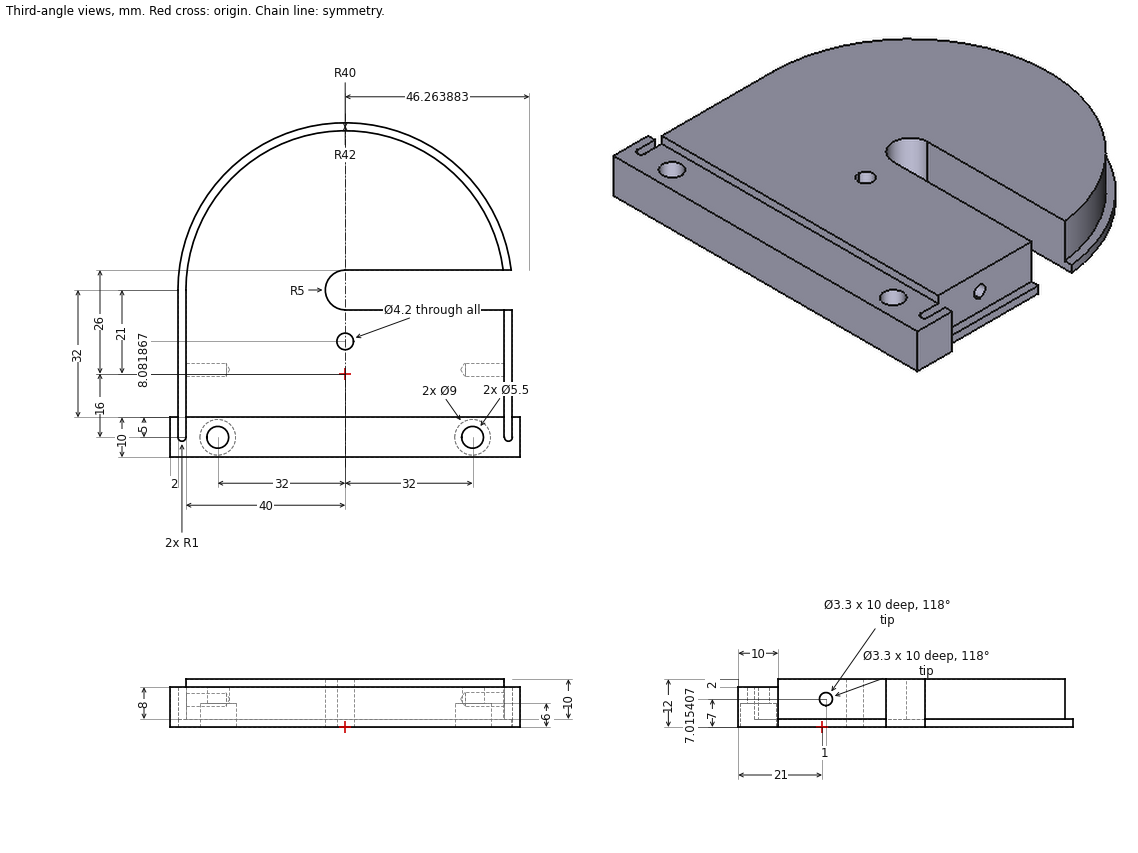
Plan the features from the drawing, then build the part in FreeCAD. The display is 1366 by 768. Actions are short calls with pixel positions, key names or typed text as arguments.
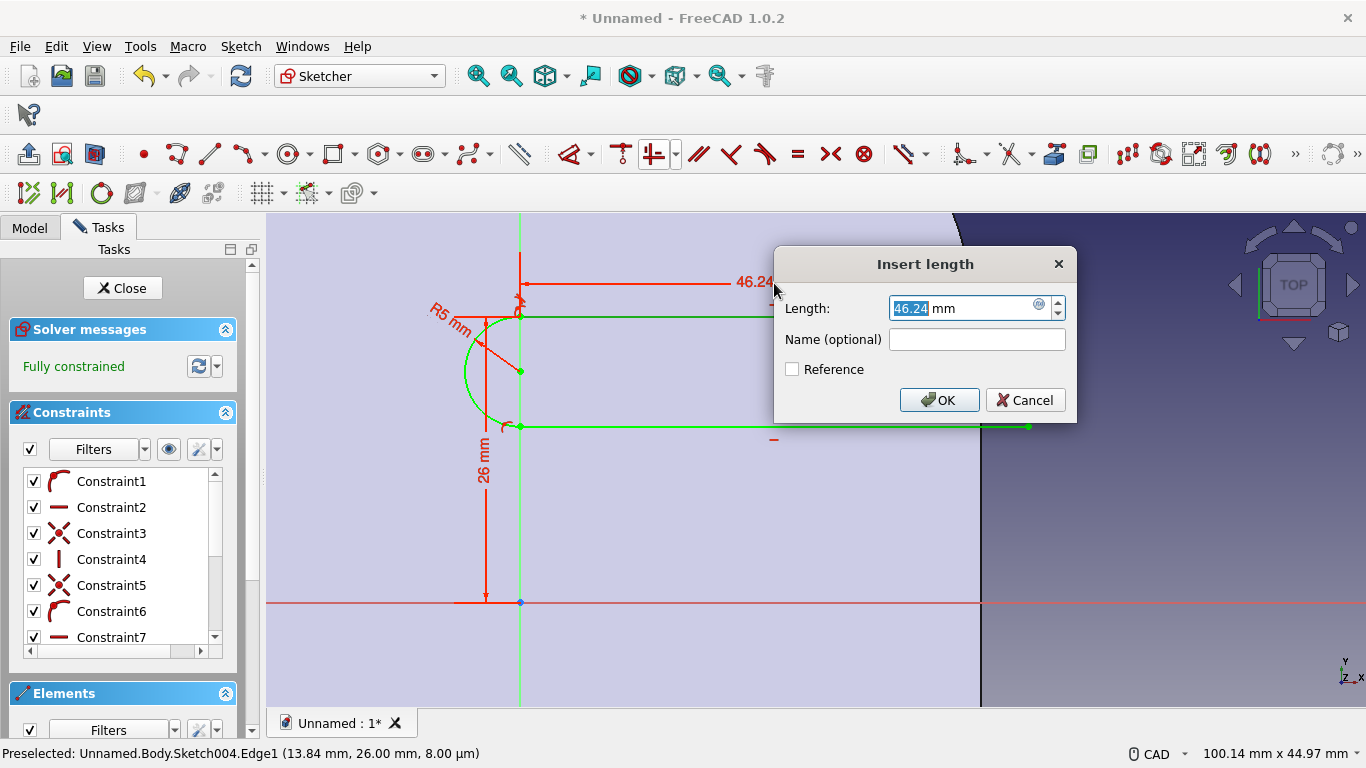
text(46.263883)
key(Return)
key(Escape)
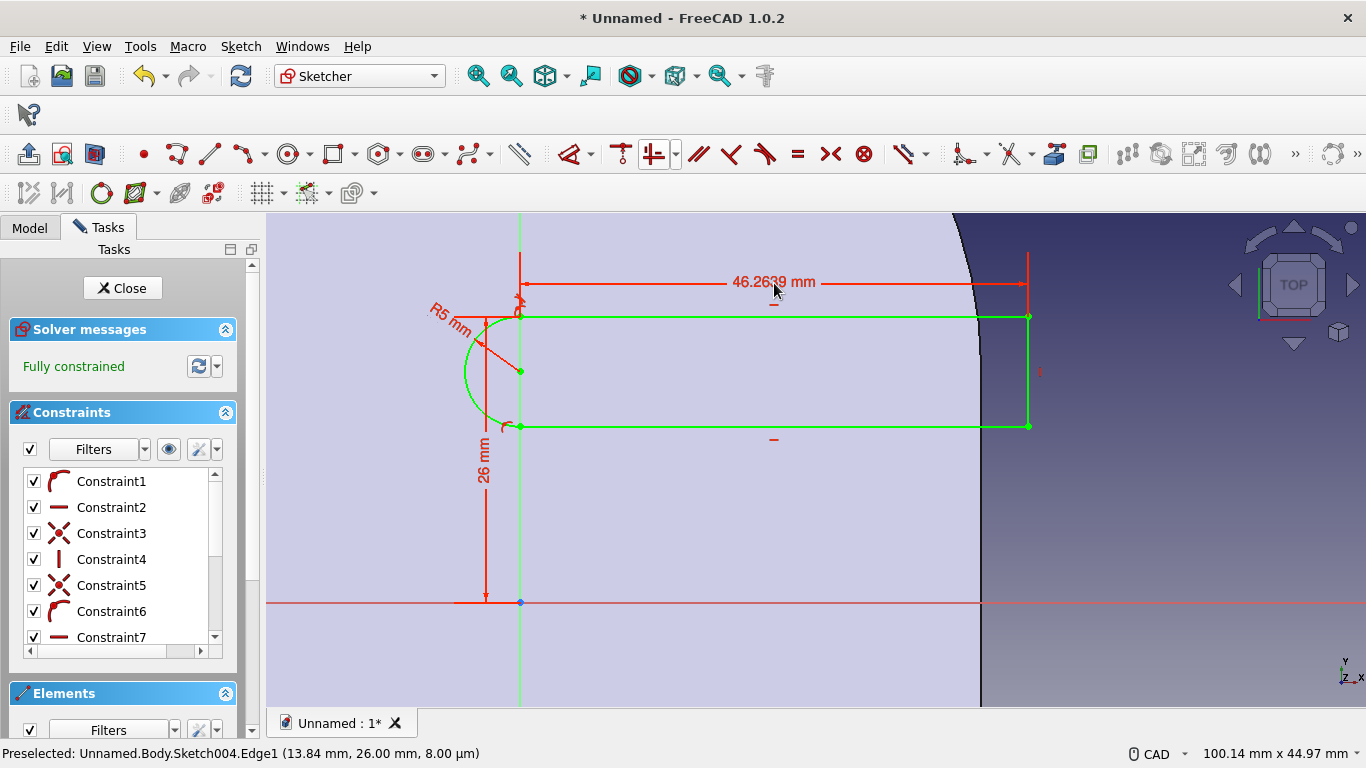
click(123, 288)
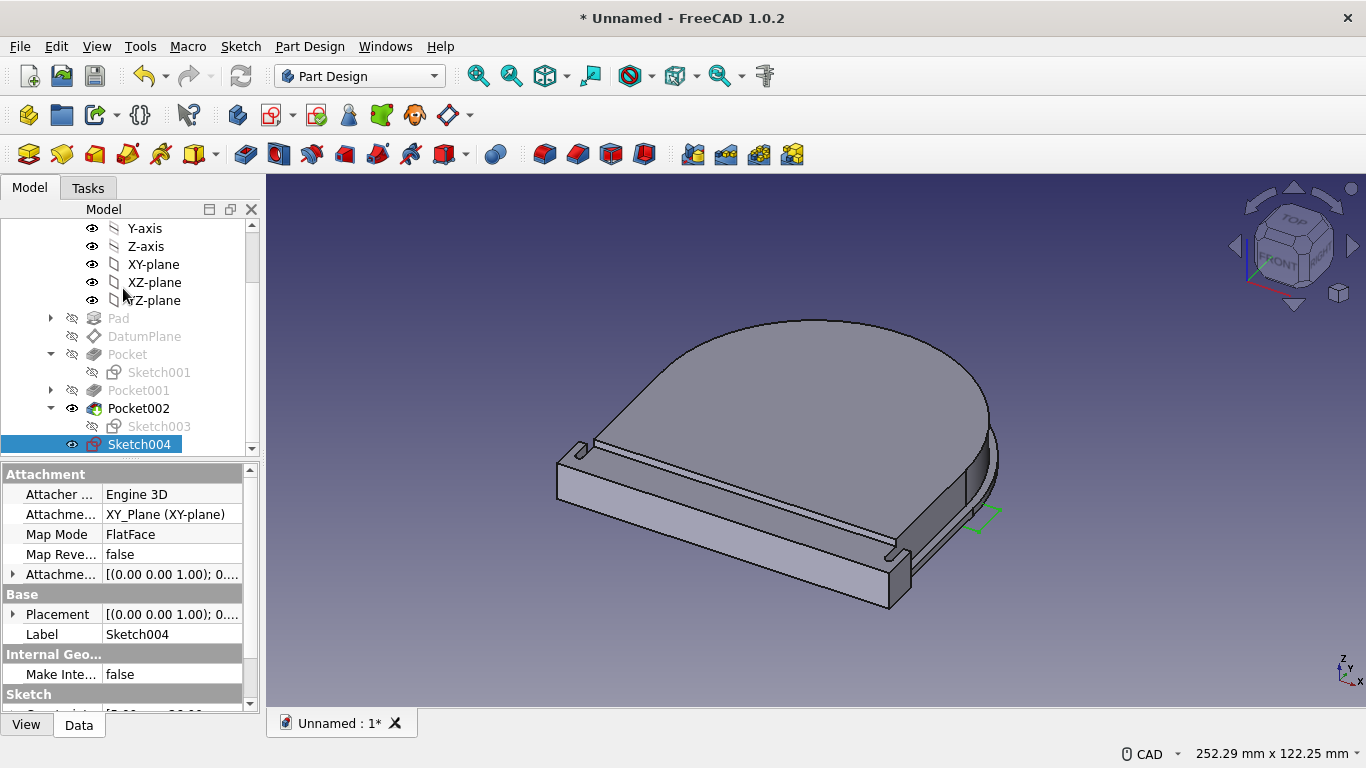
click(246, 154)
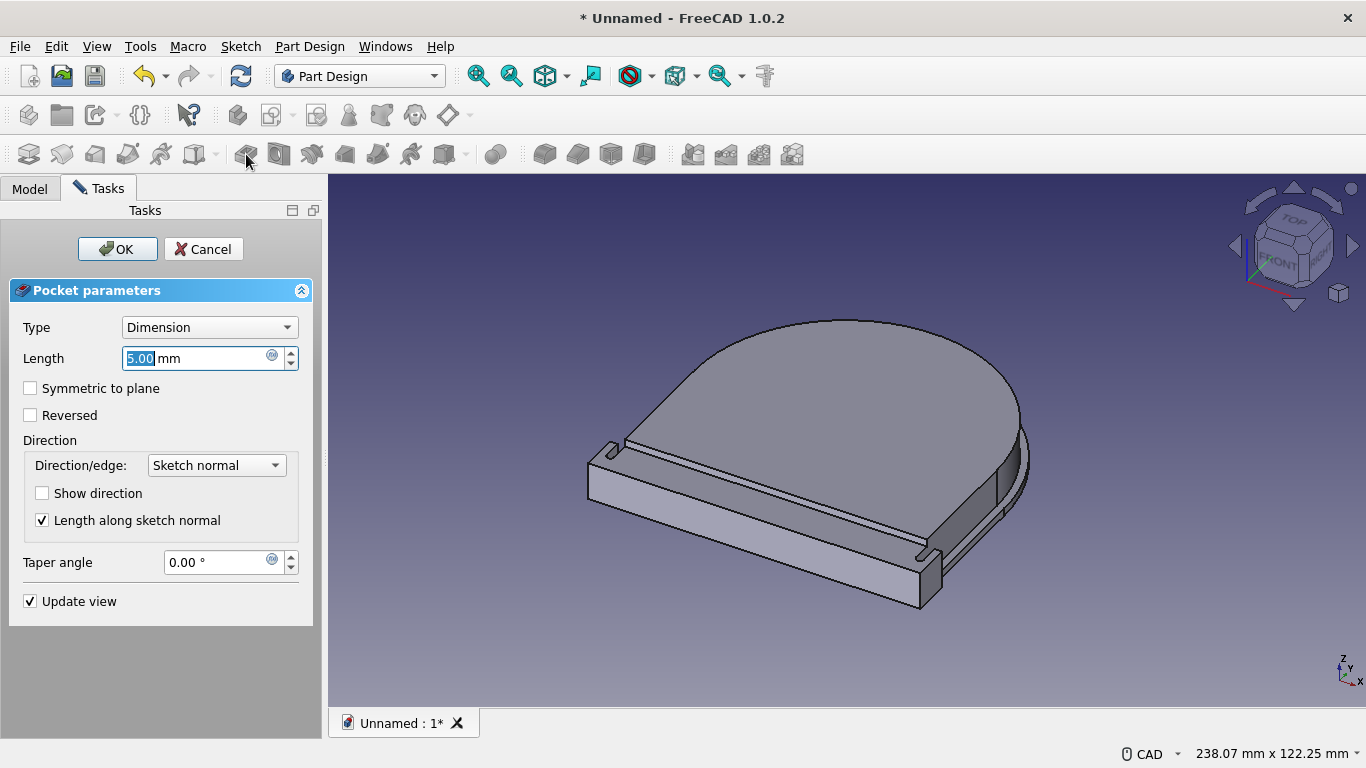
click(210, 328)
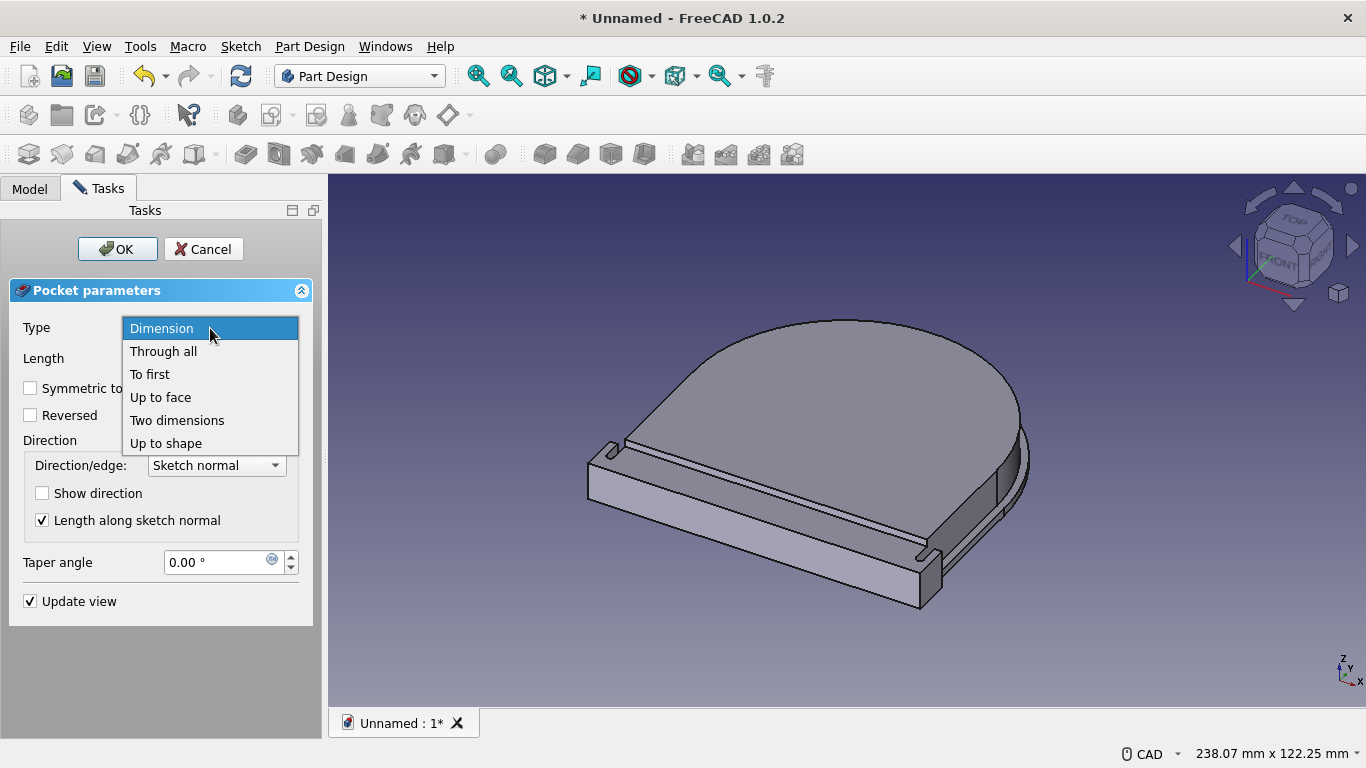
click(208, 352)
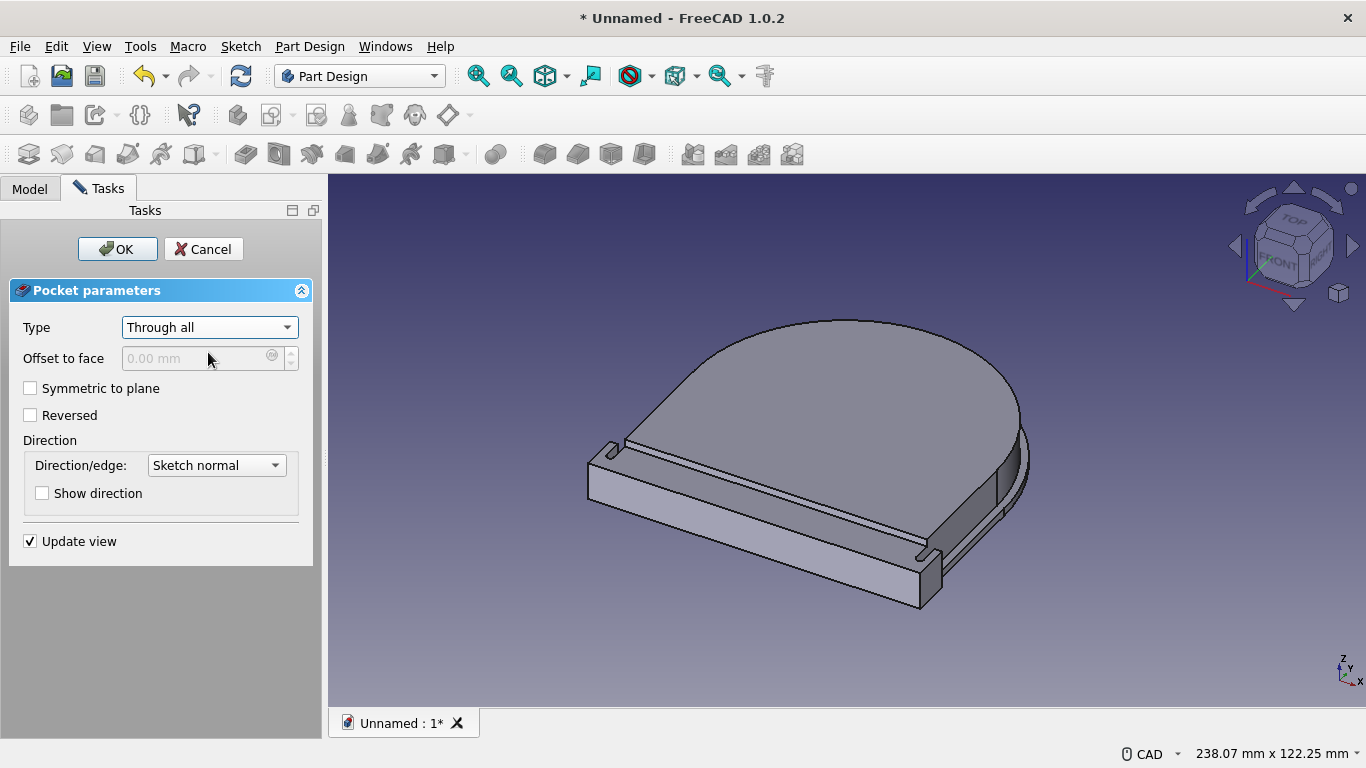
click(31, 415)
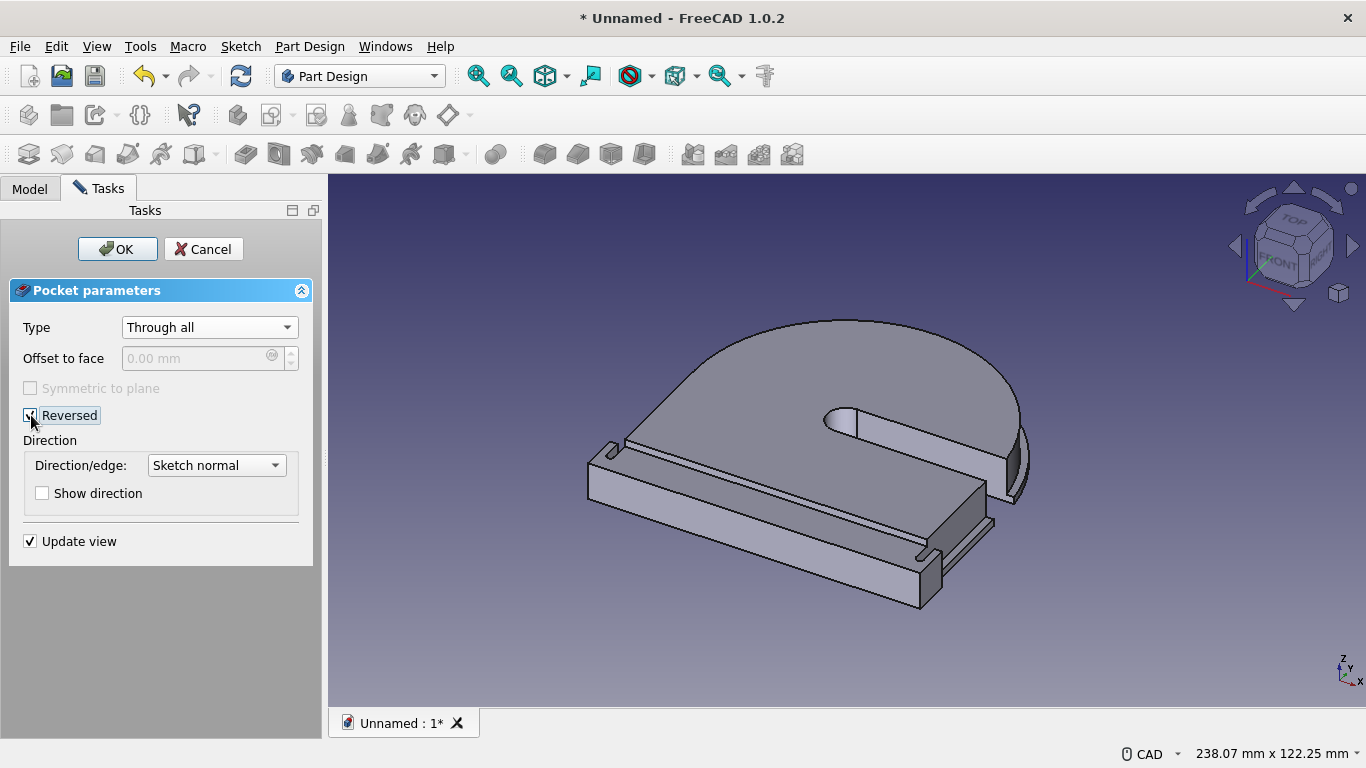
click(118, 249)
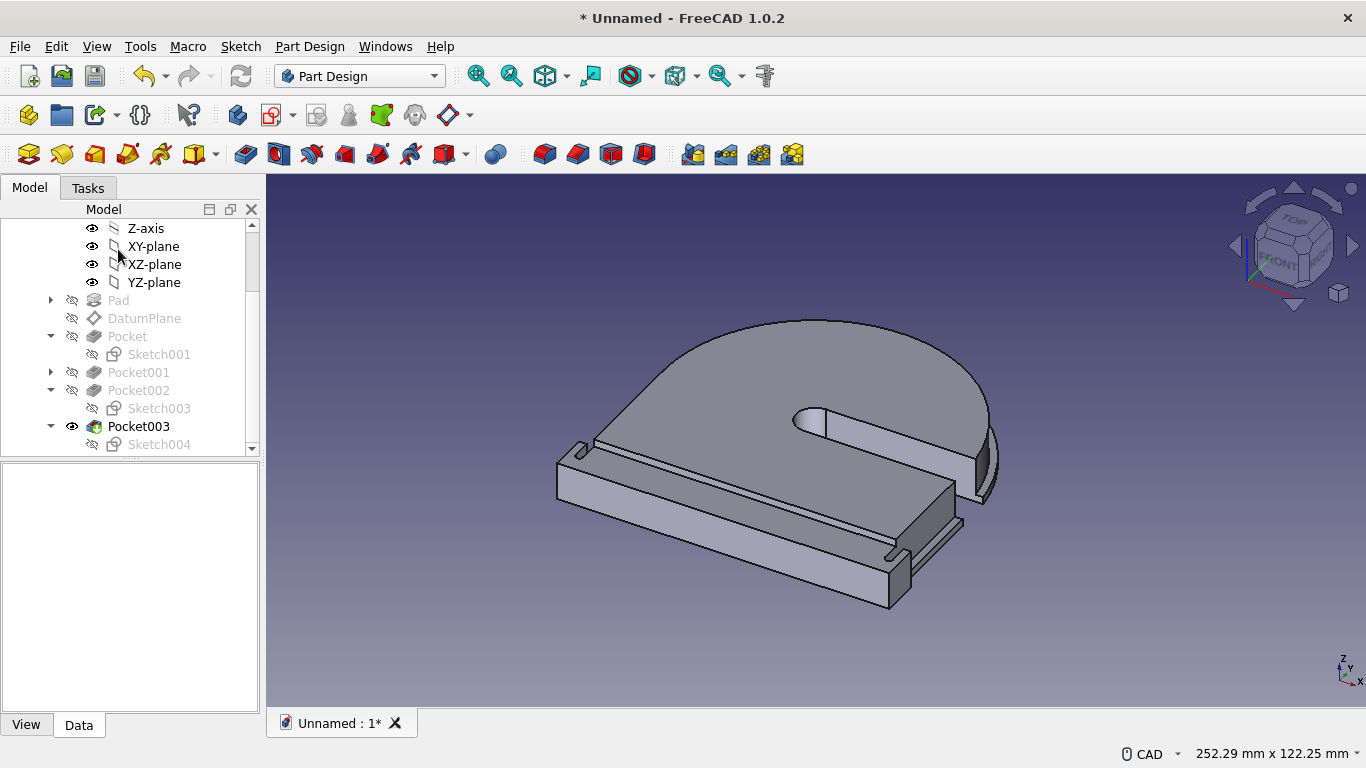
click(270, 116)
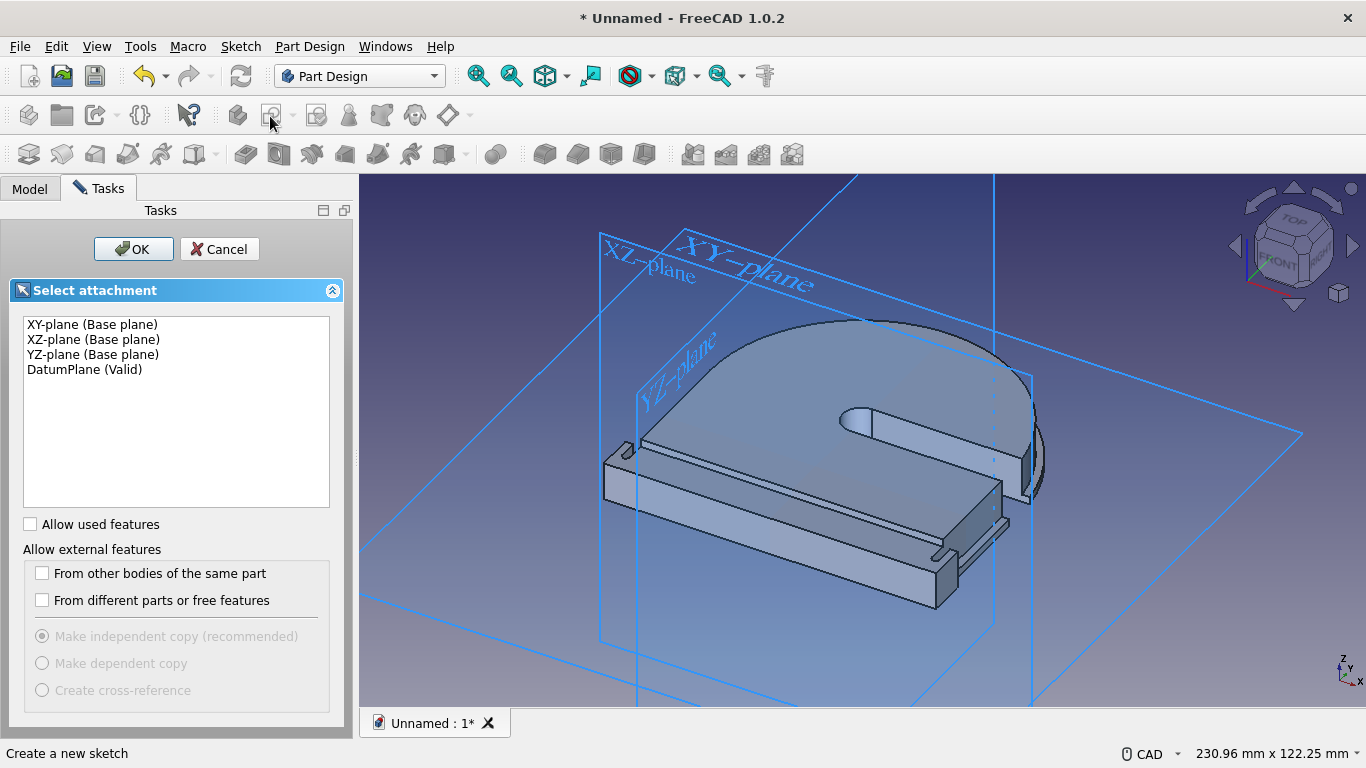
click(84, 324)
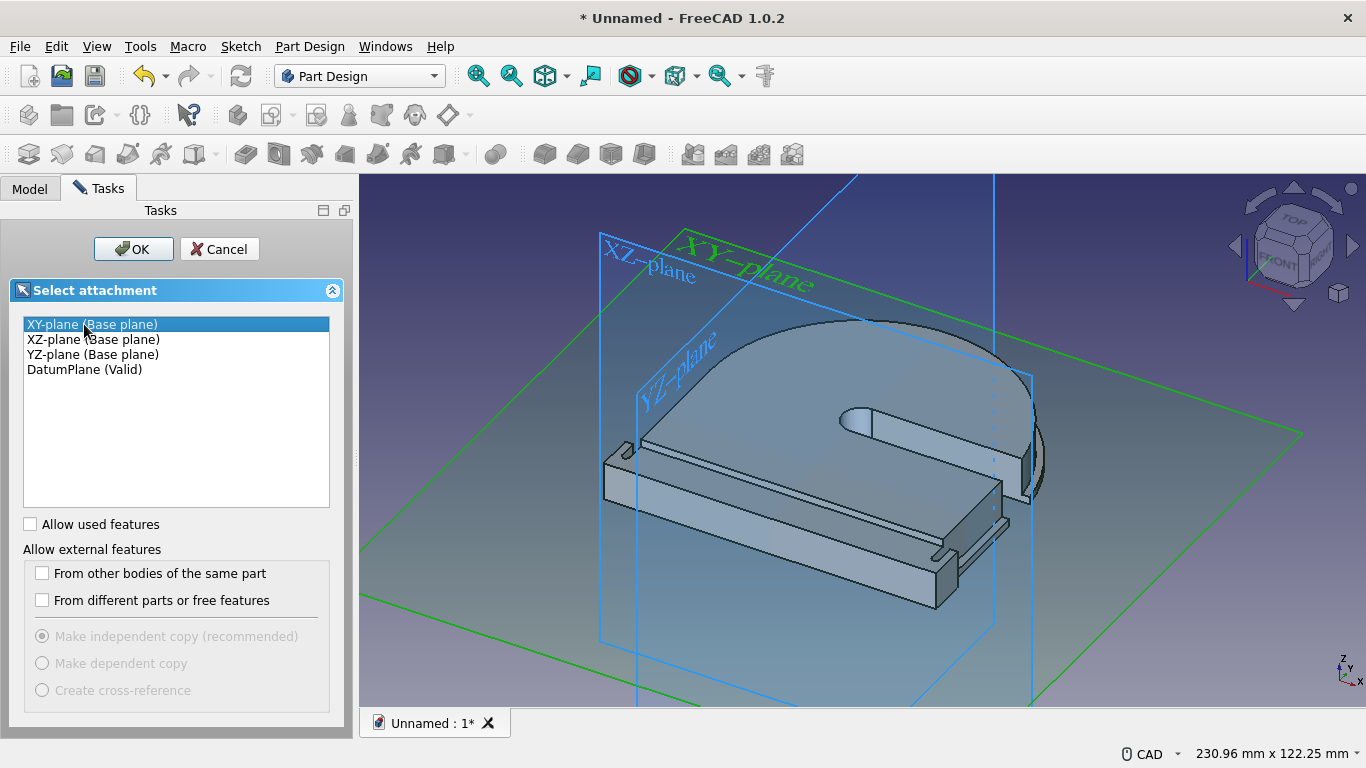
click(134, 249)